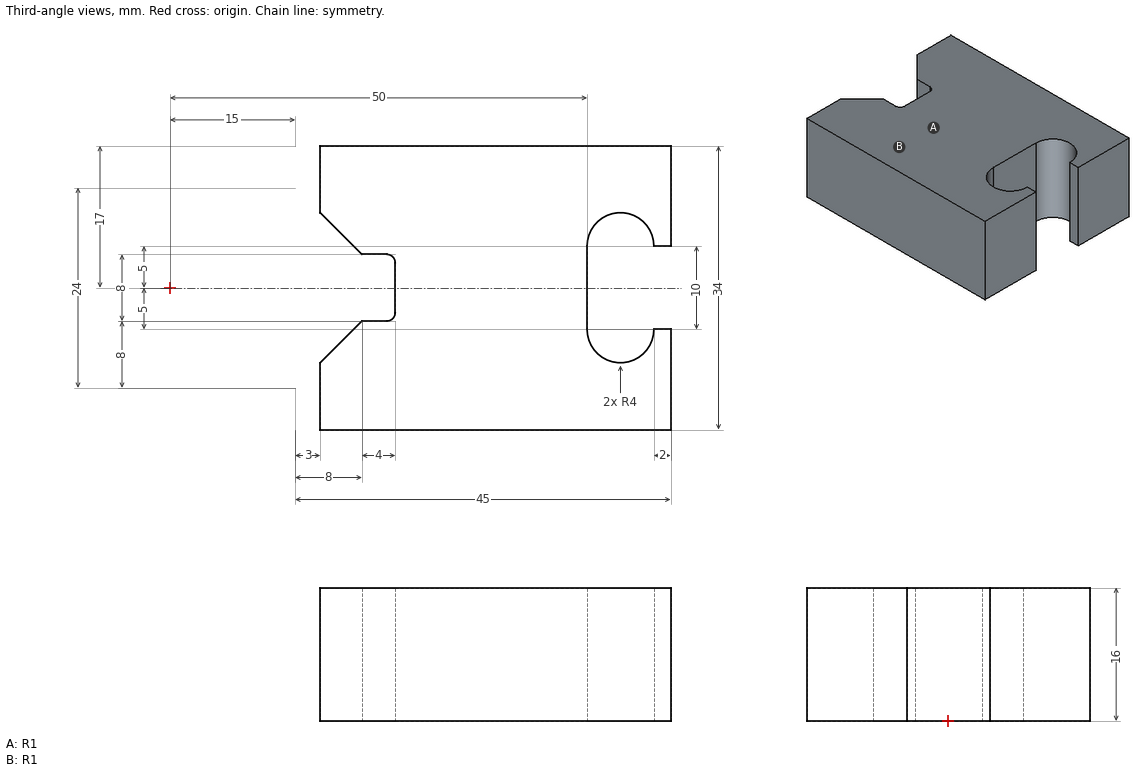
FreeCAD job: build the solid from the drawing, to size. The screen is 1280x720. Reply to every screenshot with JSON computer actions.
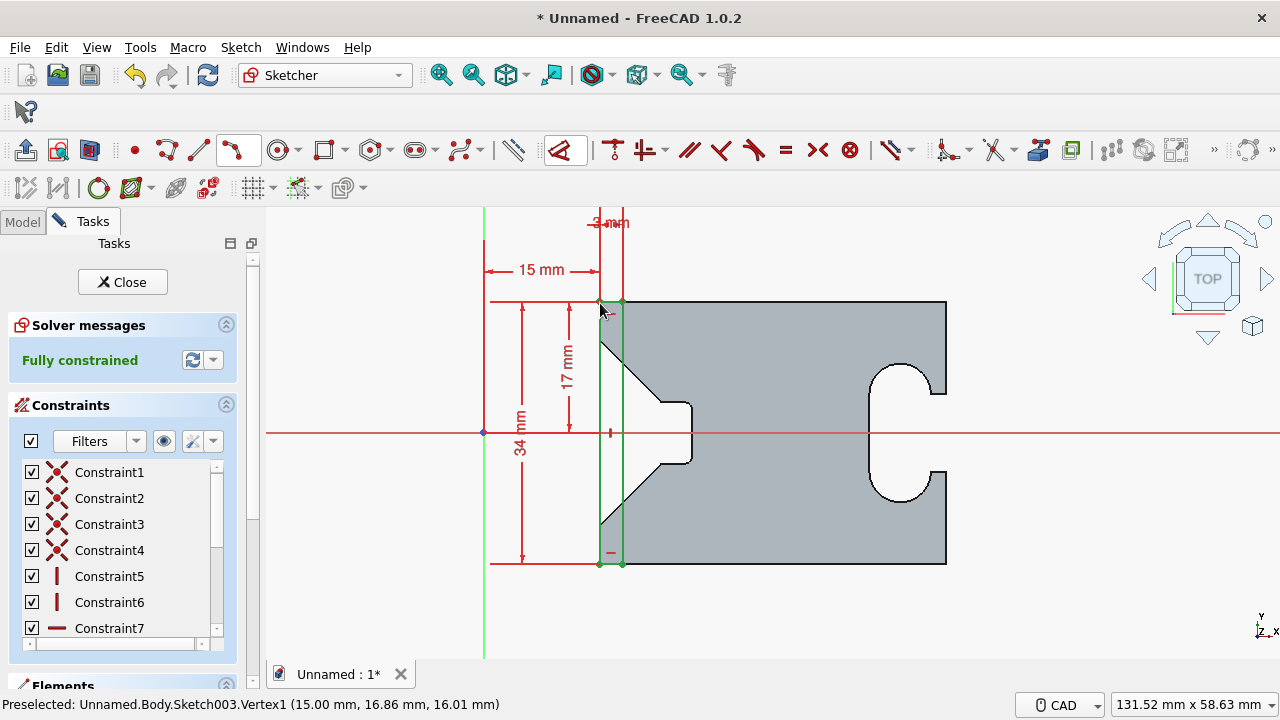
{"action": "left_click", "coordinate": [123, 282]}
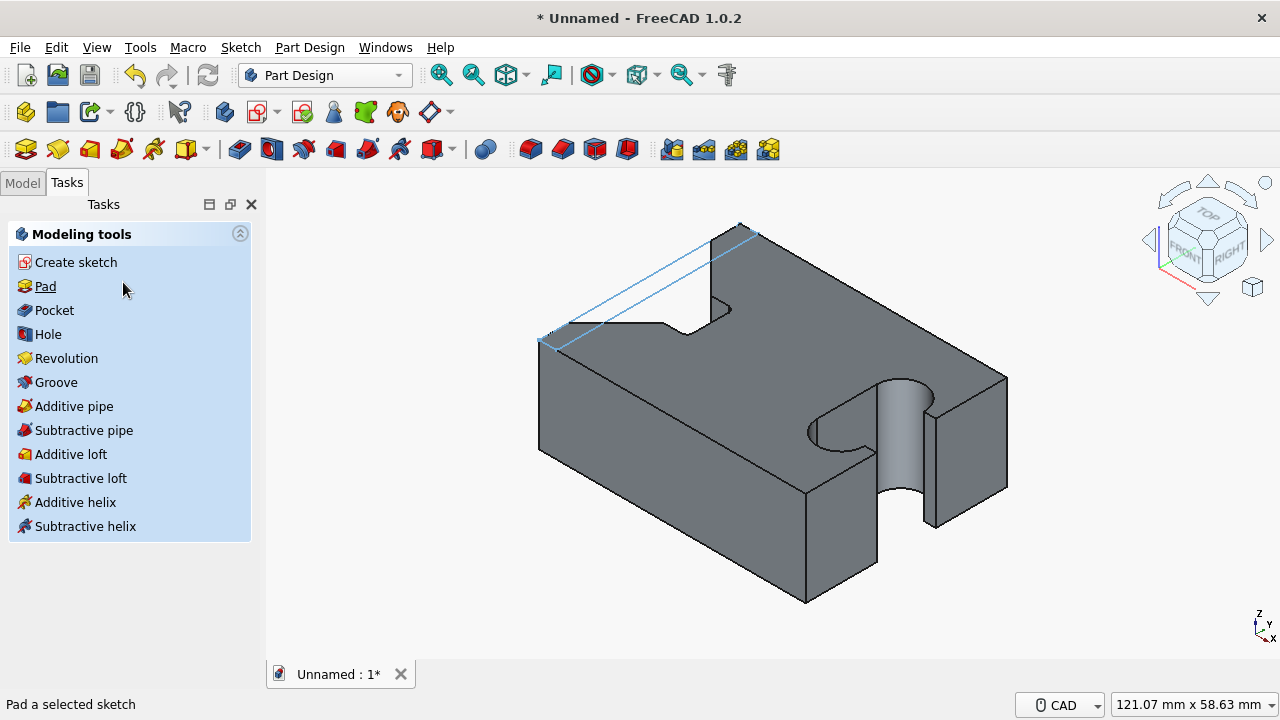
{"action": "left_click", "coordinate": [240, 150]}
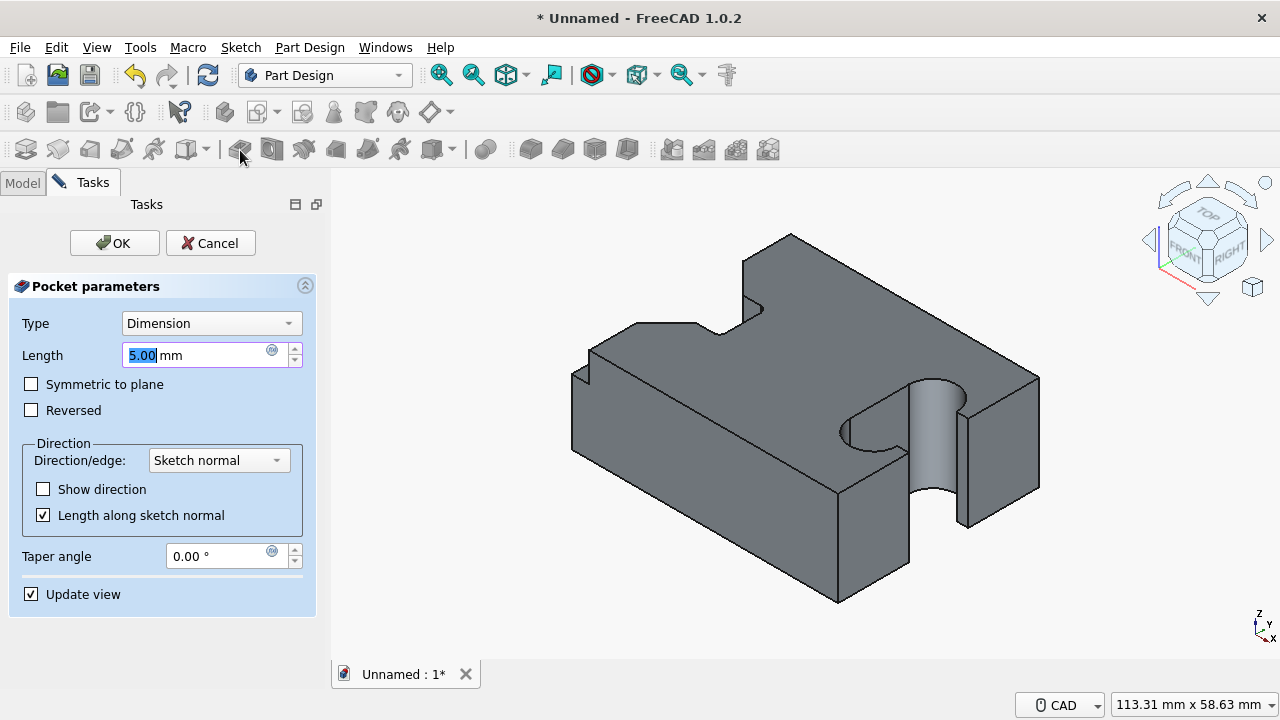
{"action": "left_click", "coordinate": [212, 324]}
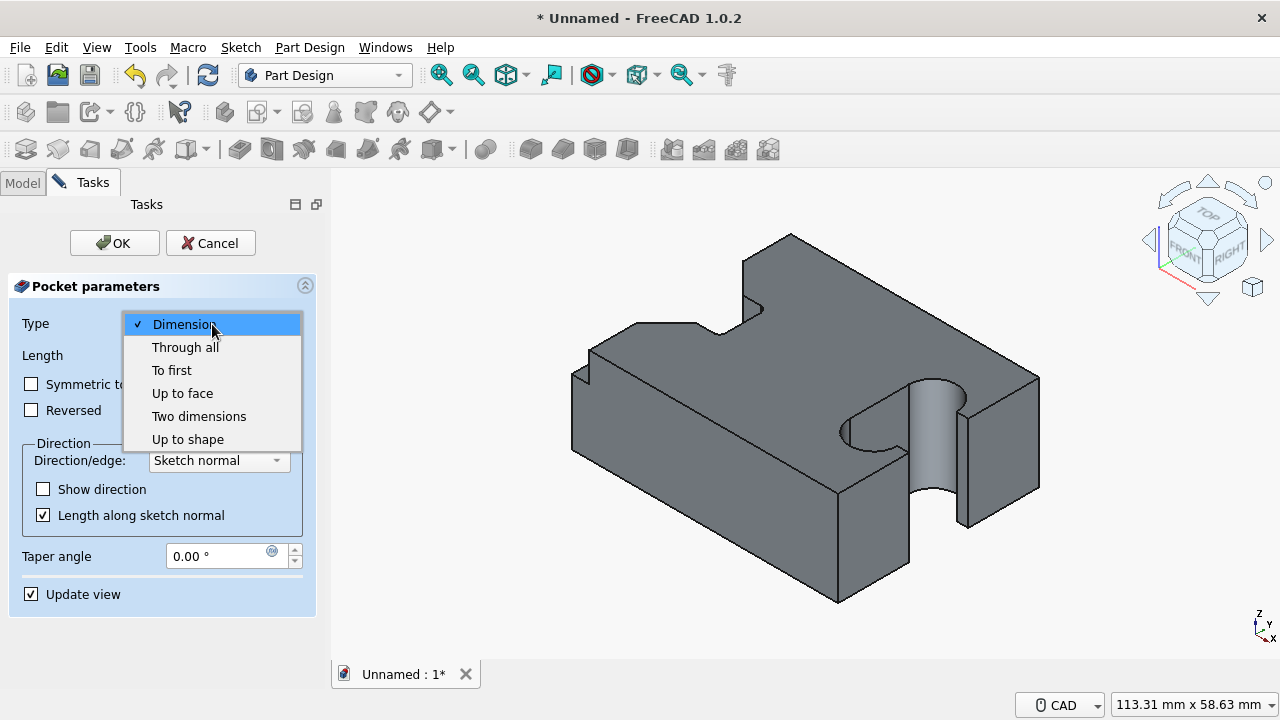
{"action": "left_click", "coordinate": [212, 348]}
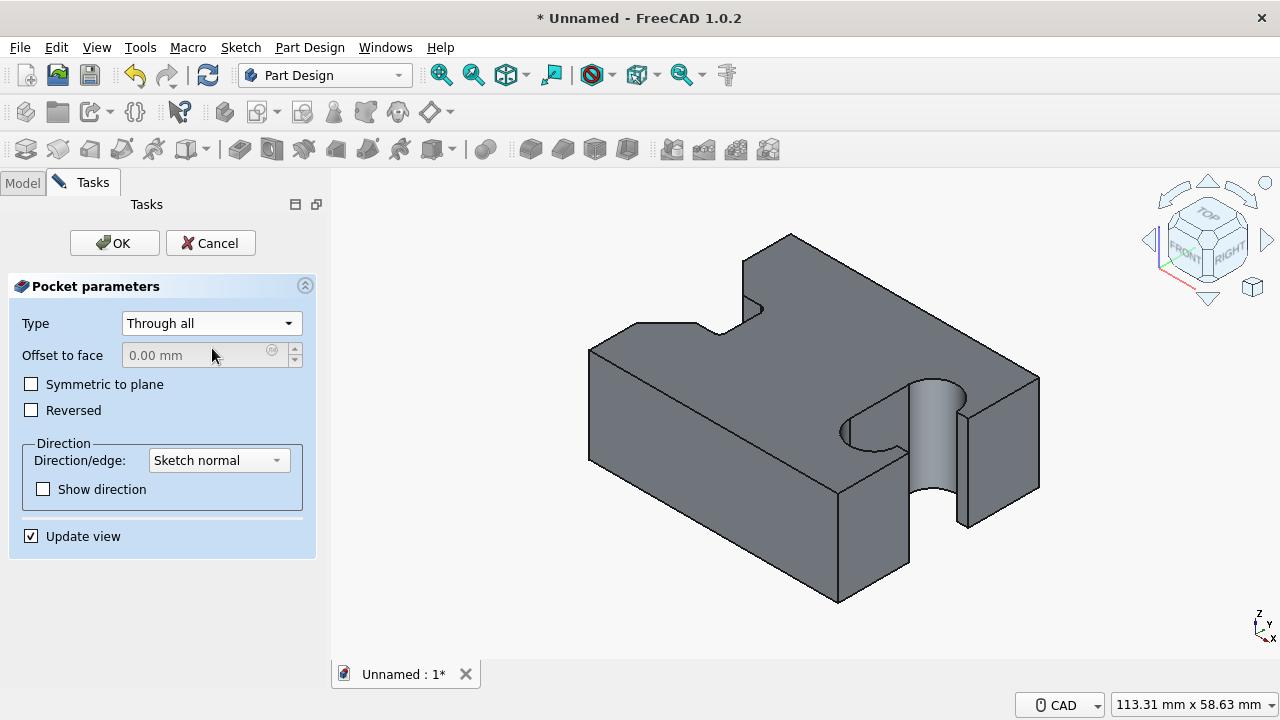
{"action": "left_click", "coordinate": [115, 243]}